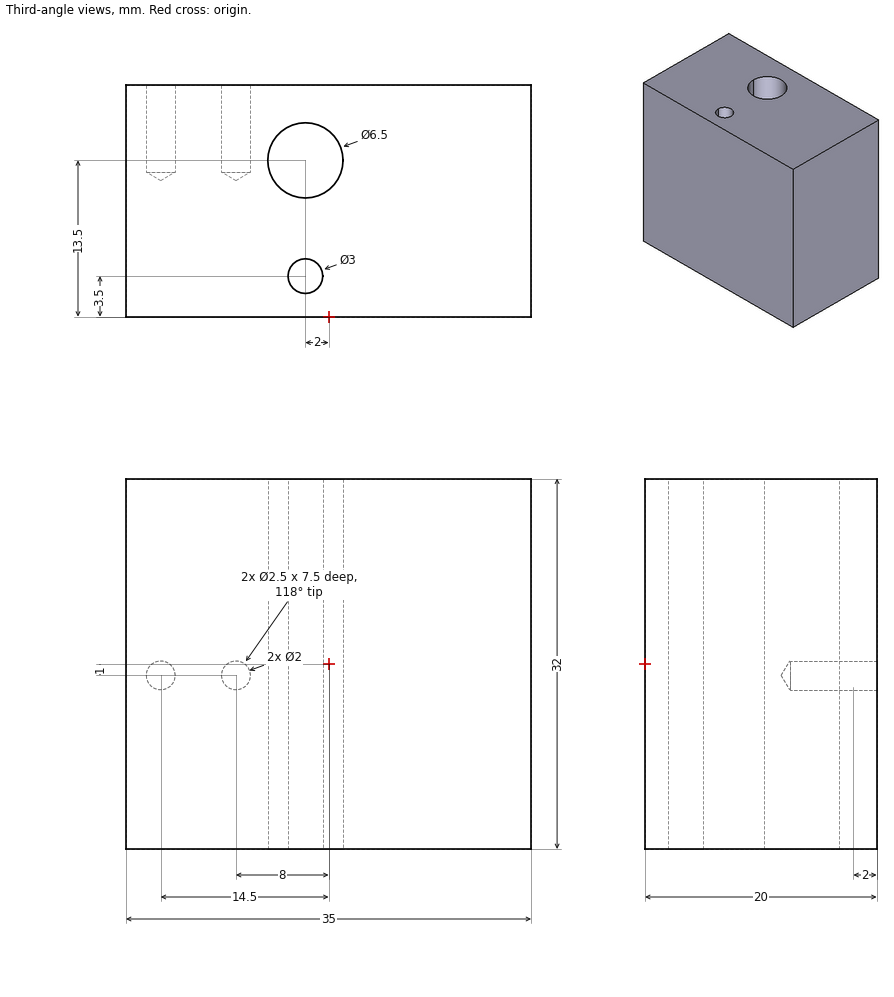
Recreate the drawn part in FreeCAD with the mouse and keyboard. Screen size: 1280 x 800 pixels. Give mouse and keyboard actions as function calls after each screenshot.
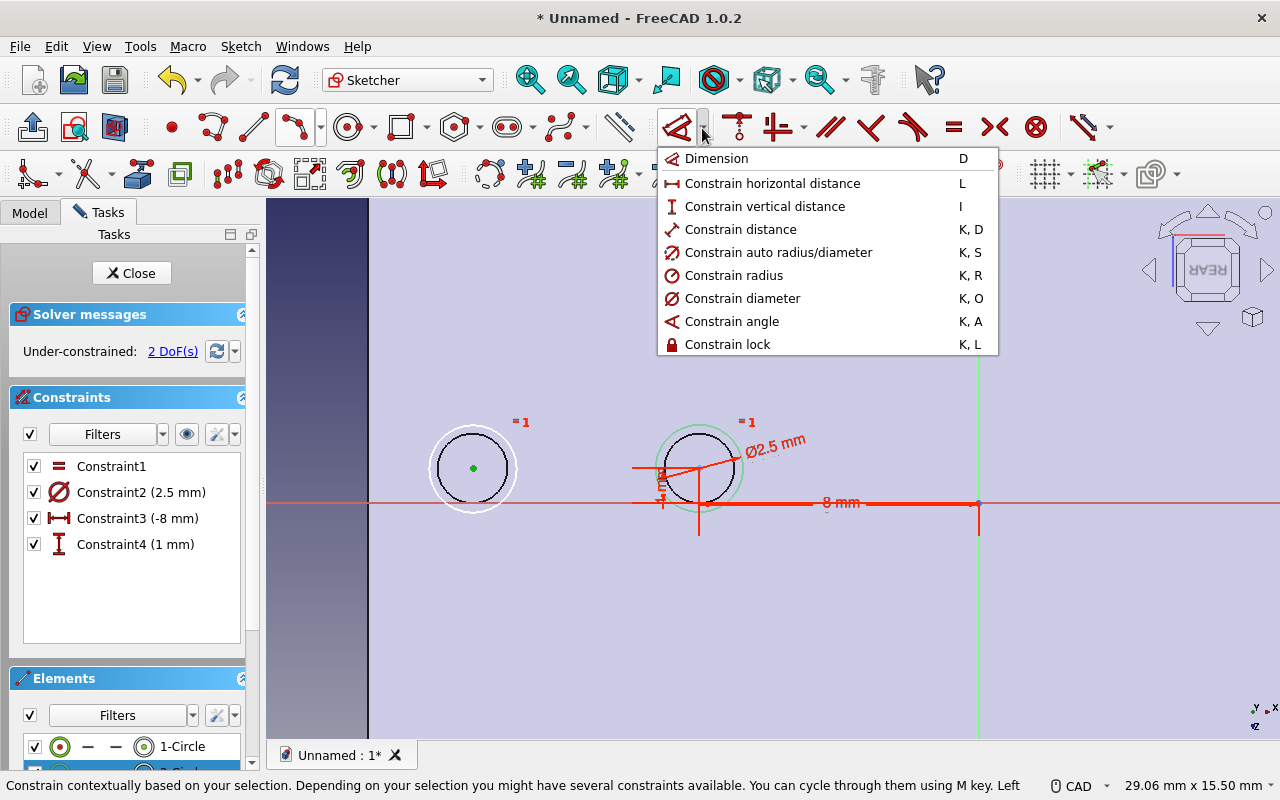
click(828, 206)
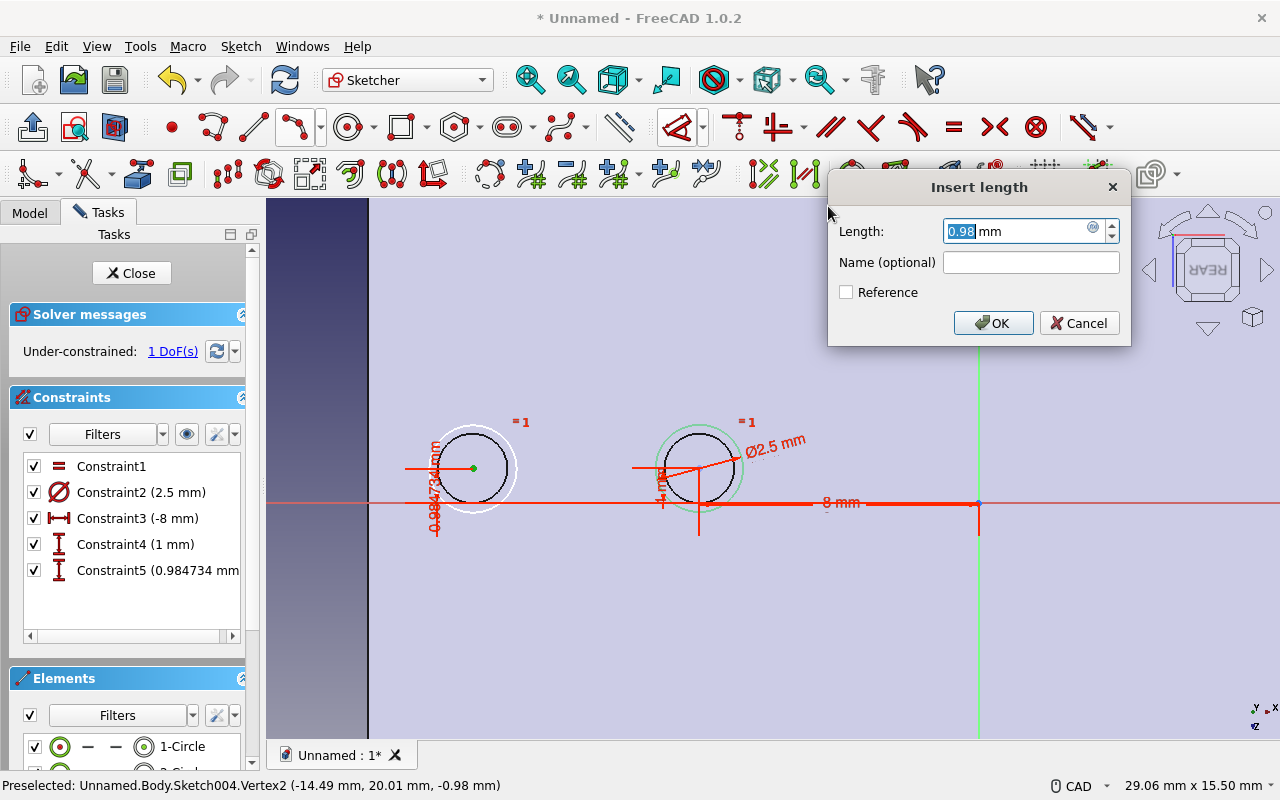
text(1)
key(Return)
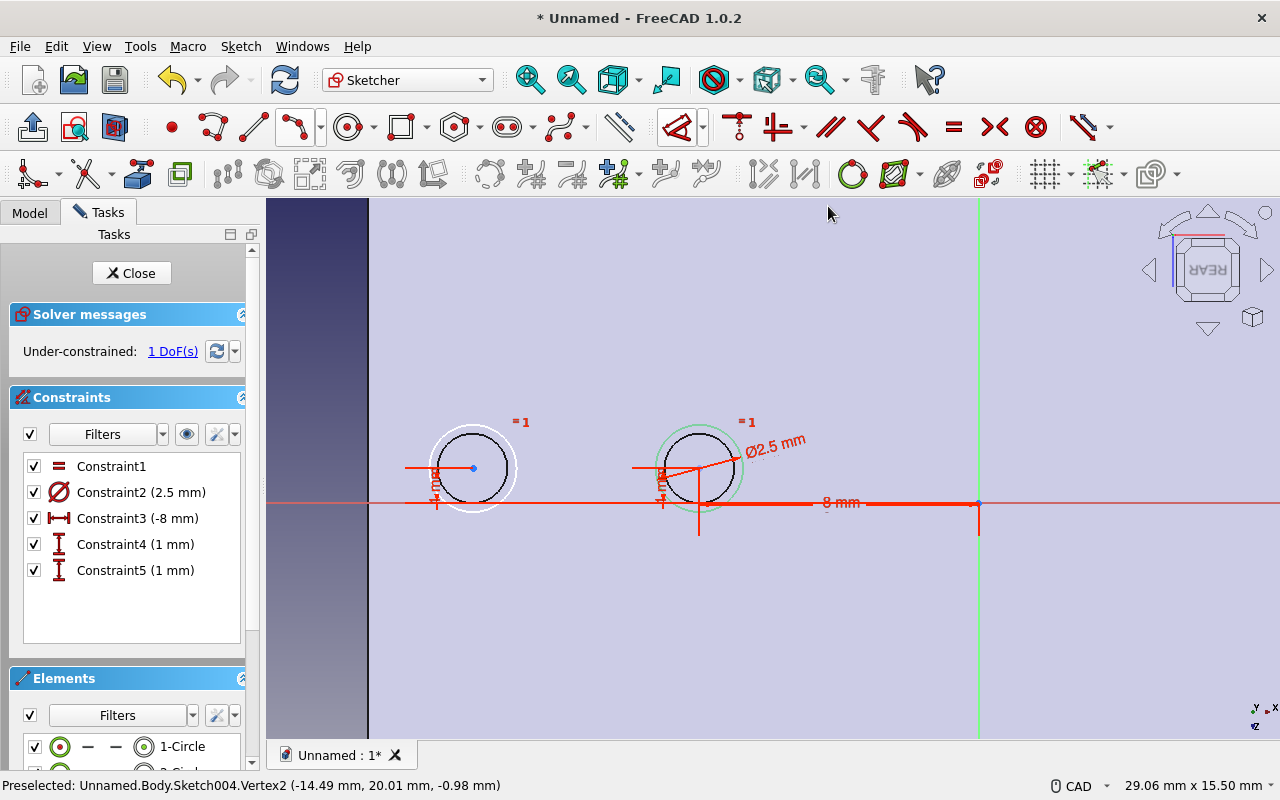
click(473, 468)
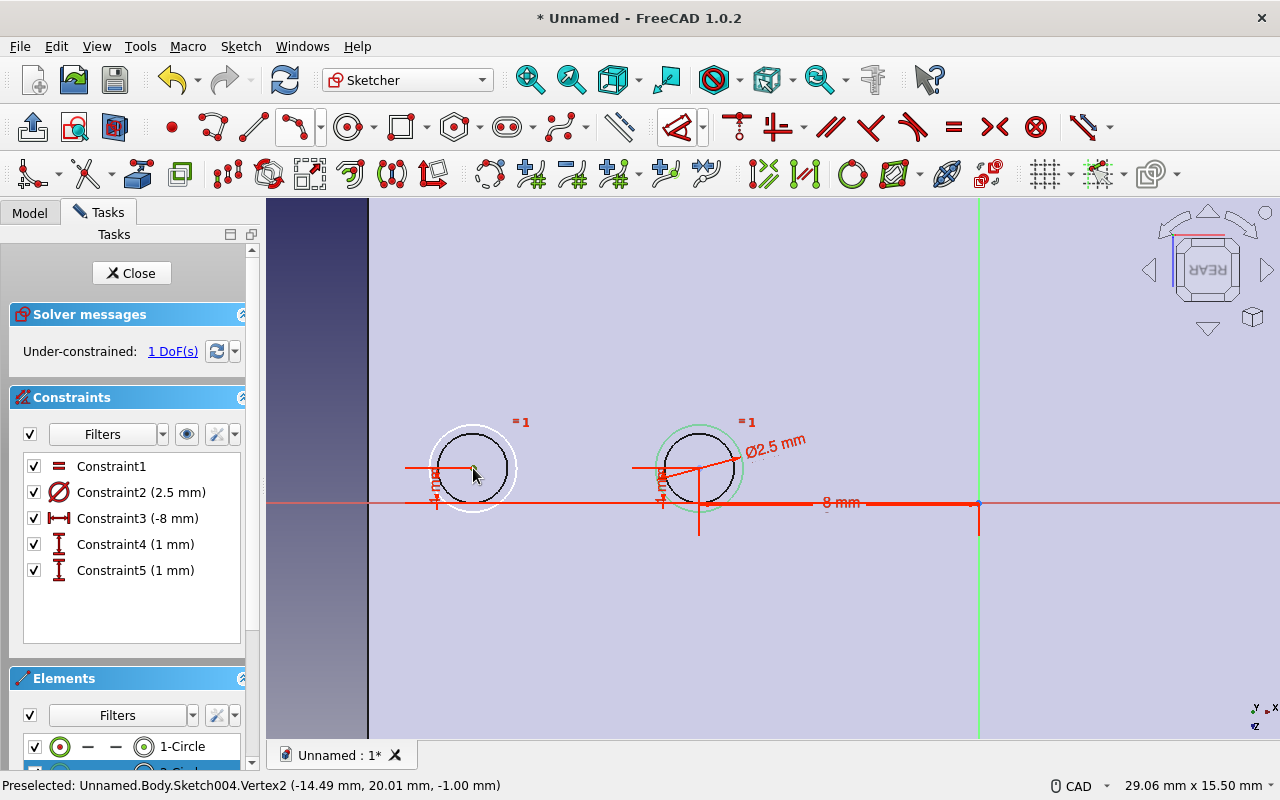
key(l)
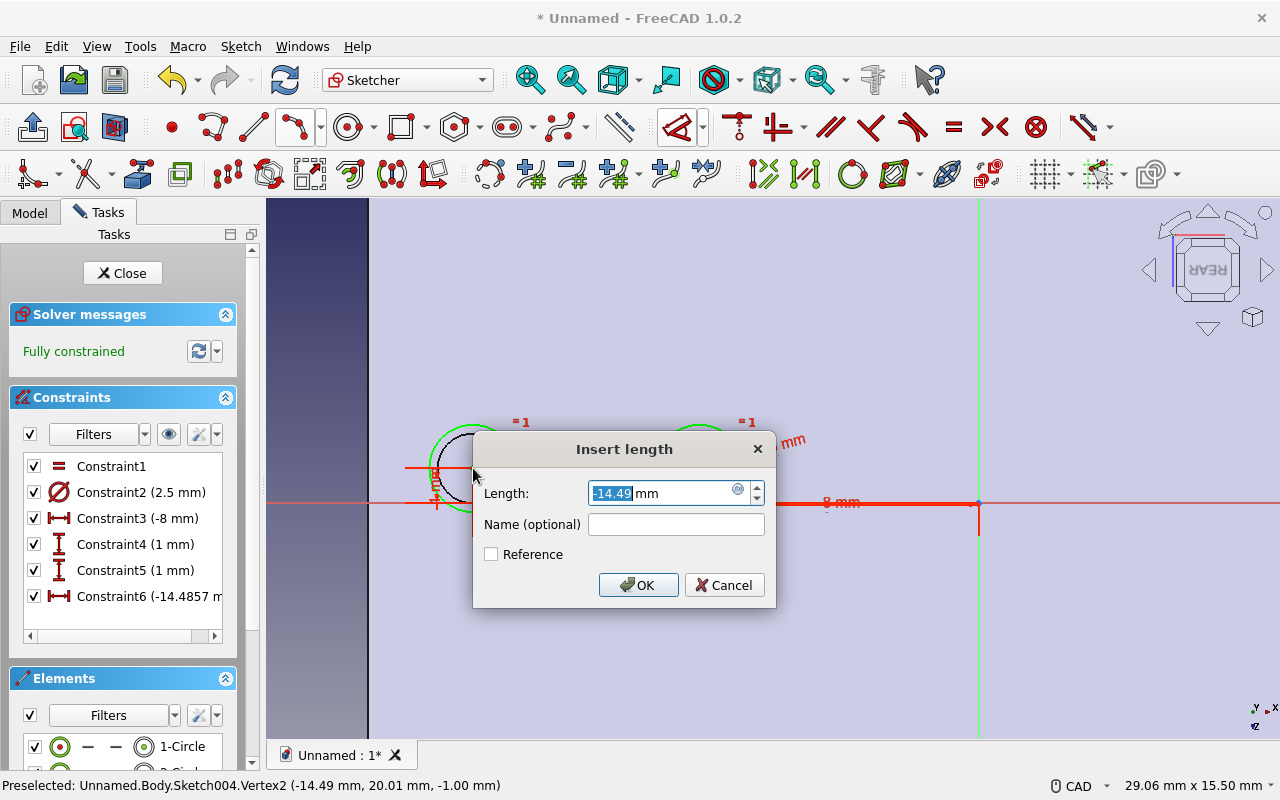
text(-14.5)
key(Return)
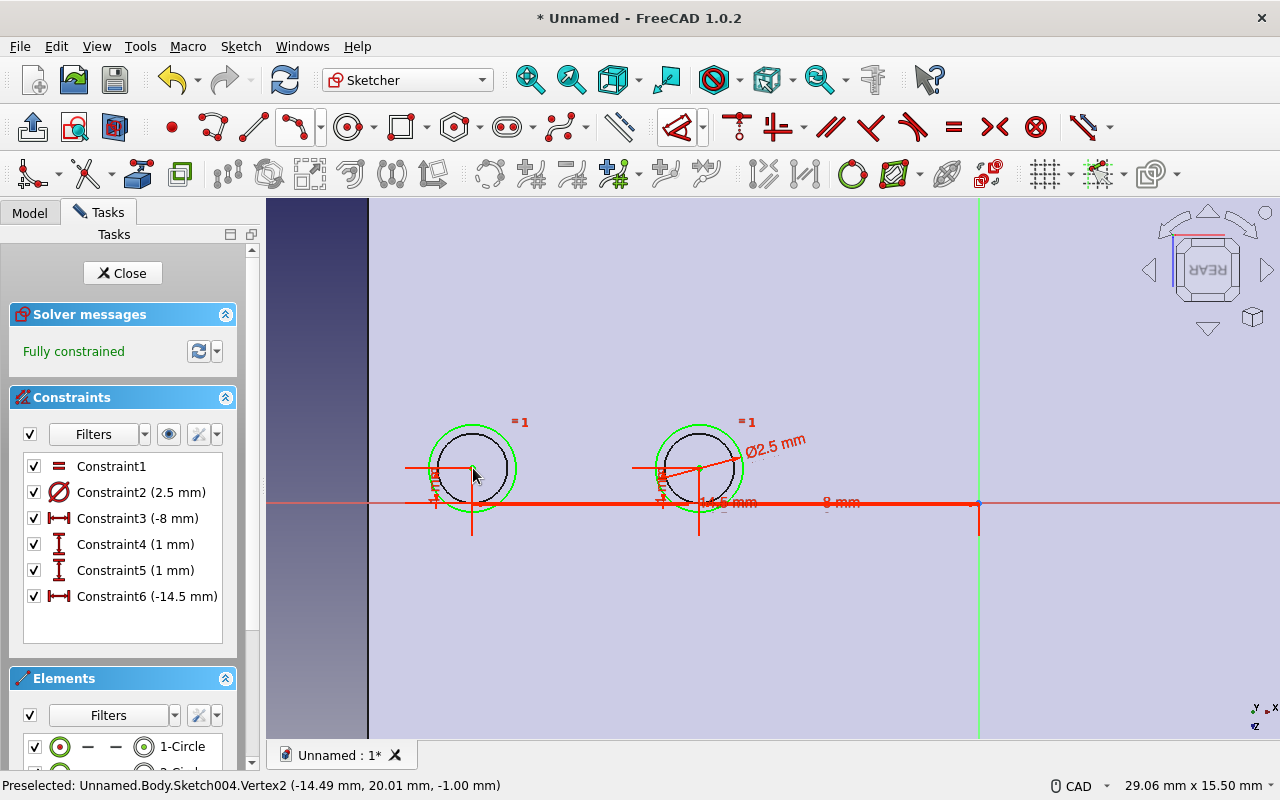
click(123, 273)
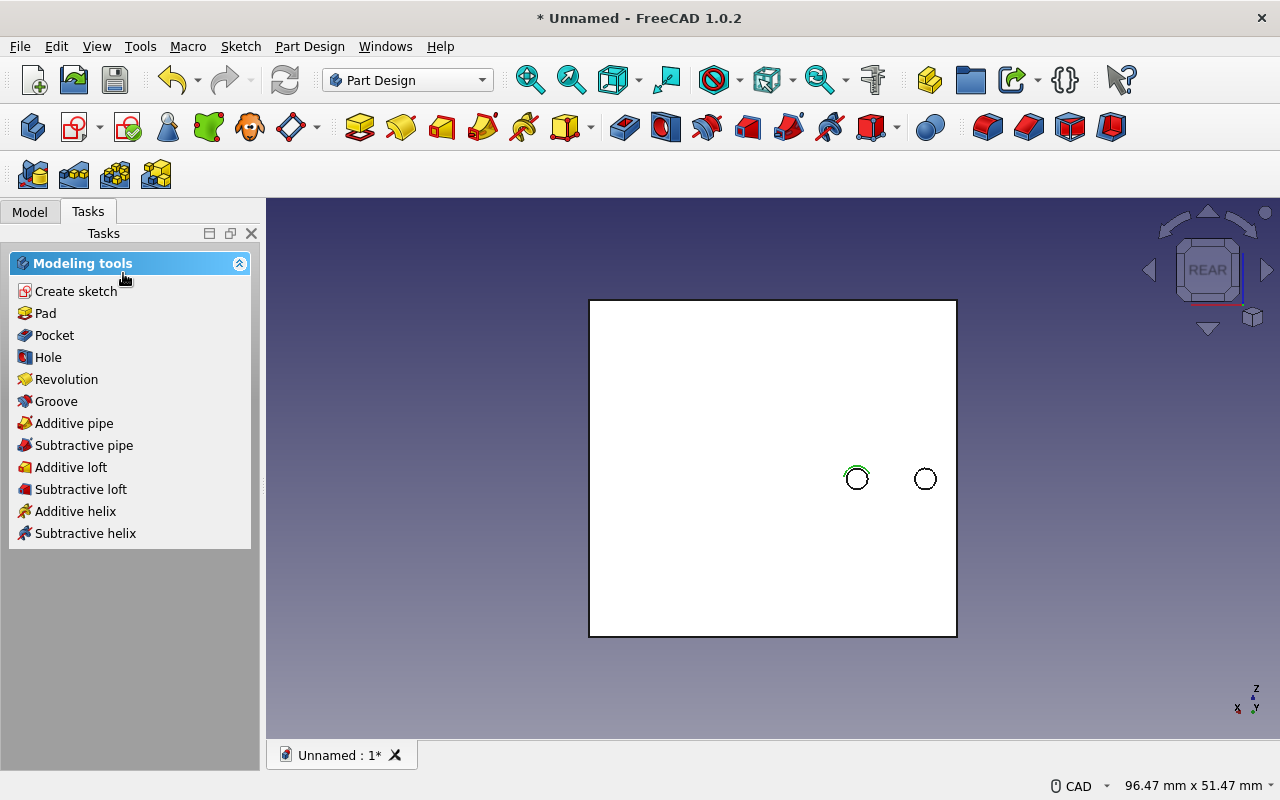
click(666, 128)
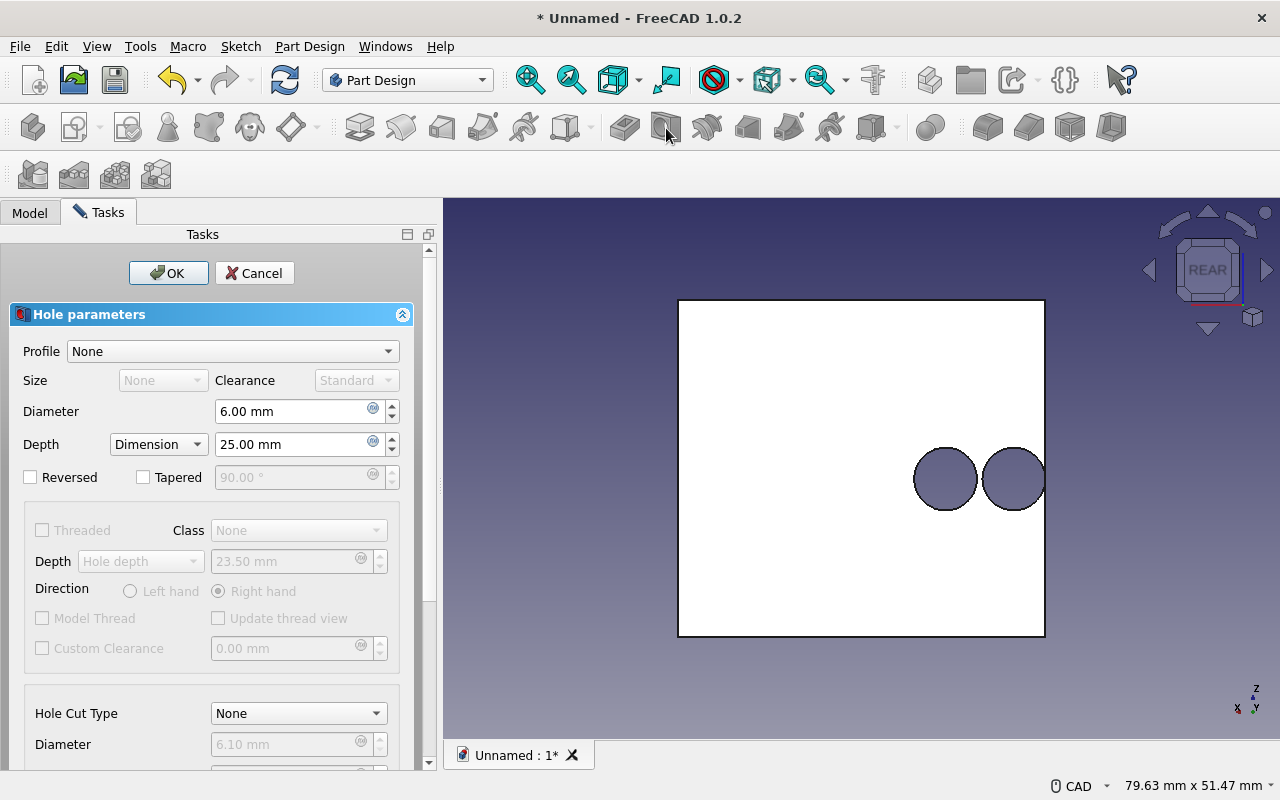
triple_click(300, 412)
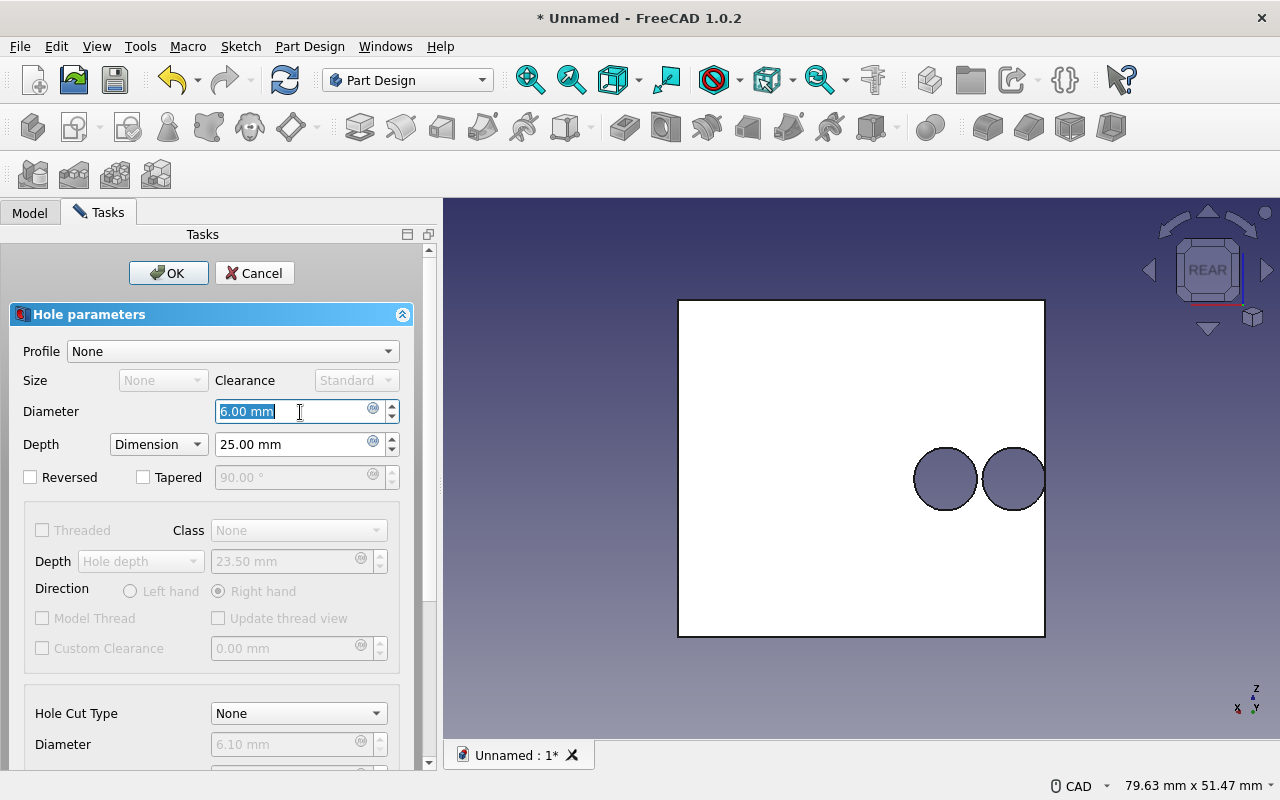
text(2.5)
key(Tab)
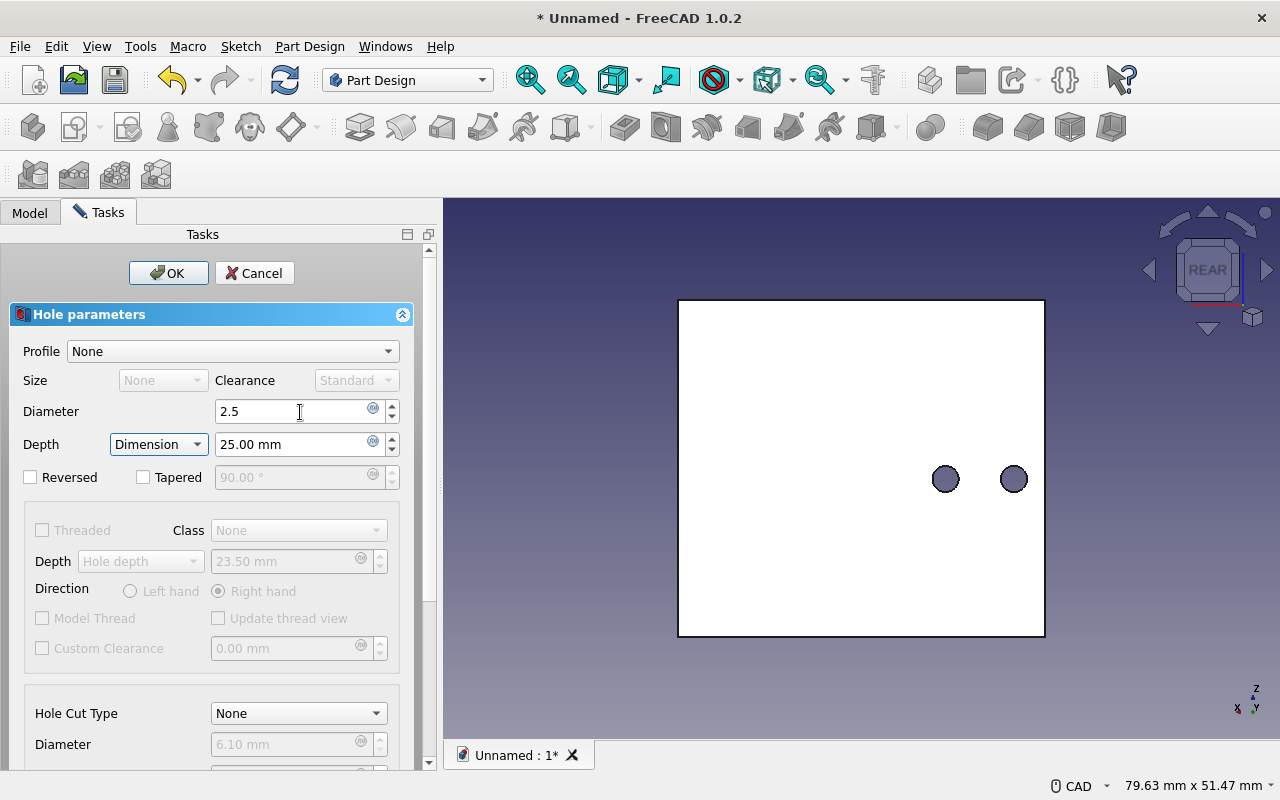
triple_click(300, 444)